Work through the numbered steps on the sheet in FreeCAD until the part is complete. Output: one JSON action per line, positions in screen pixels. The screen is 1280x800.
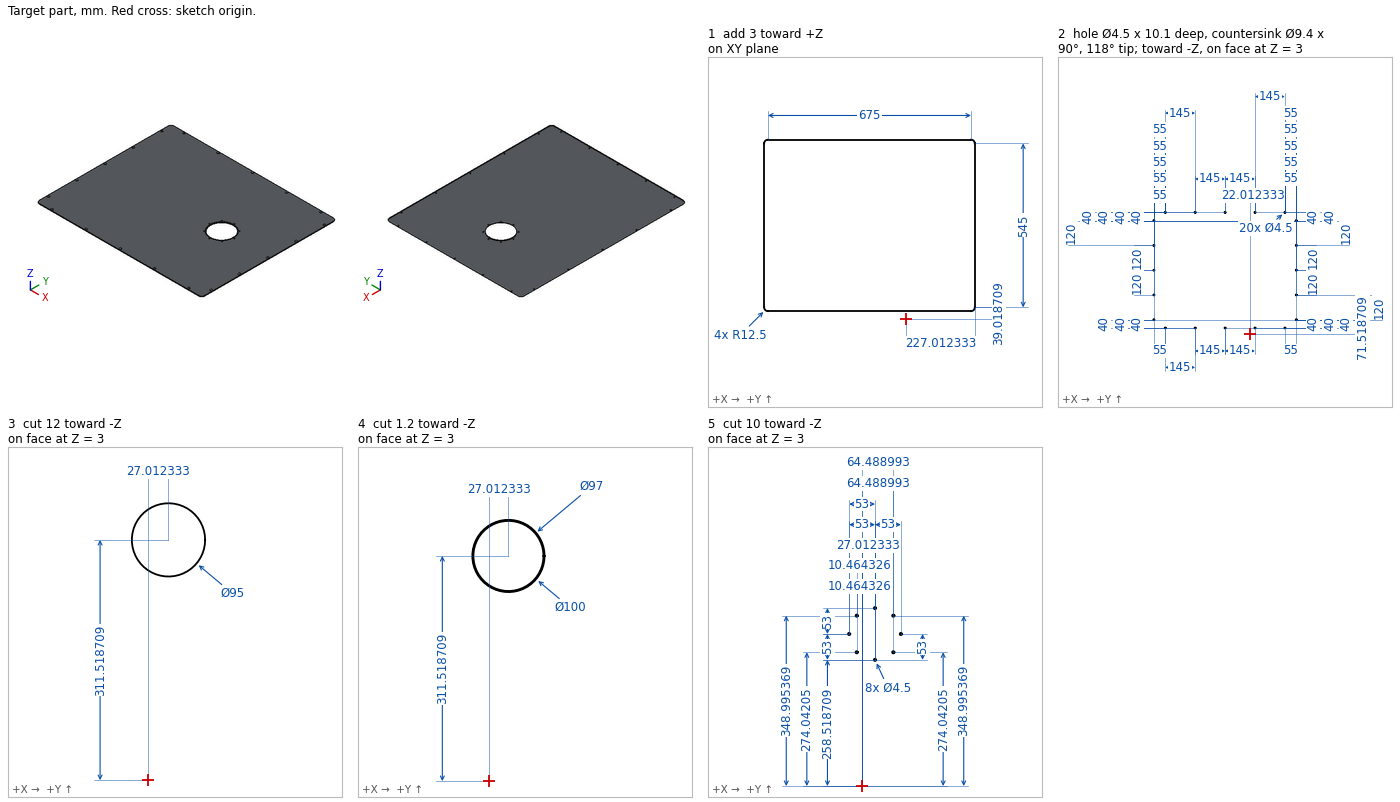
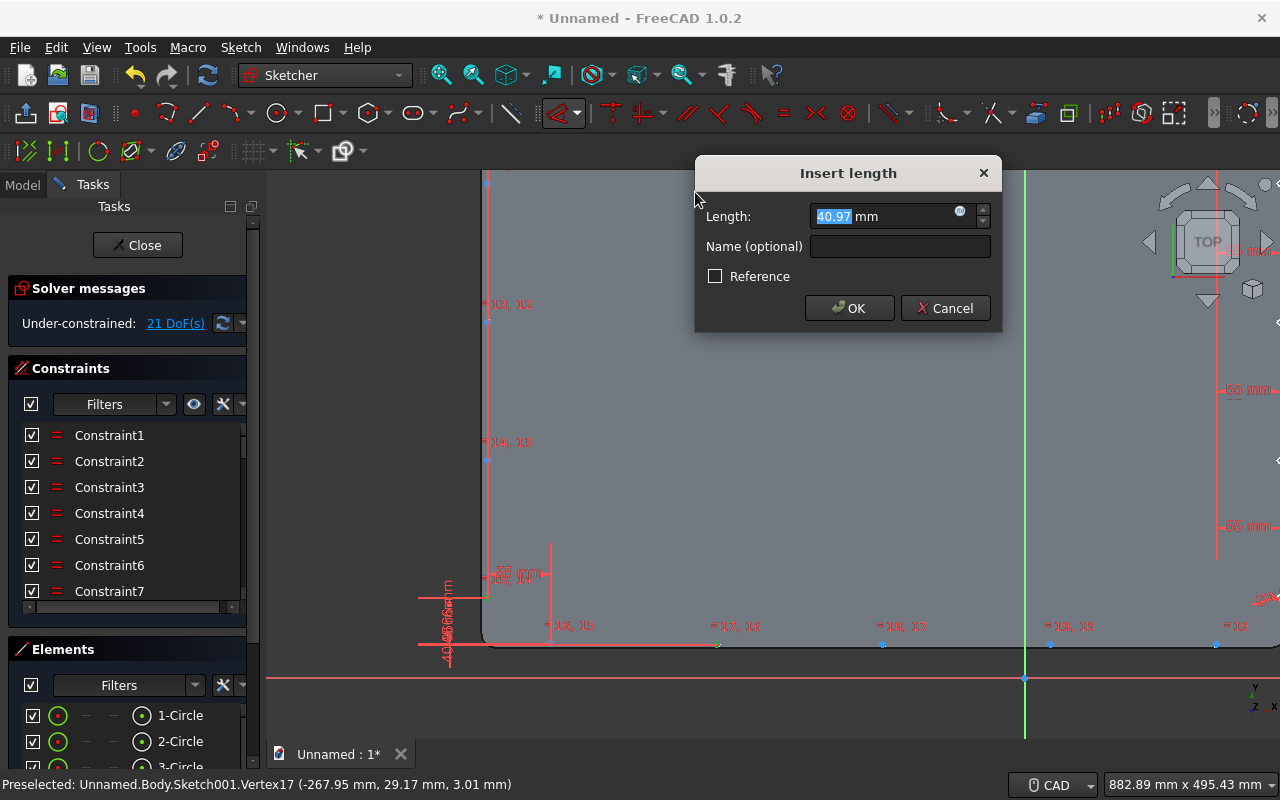
{"action": "type", "text": "40"}
{"action": "key", "text": "Return"}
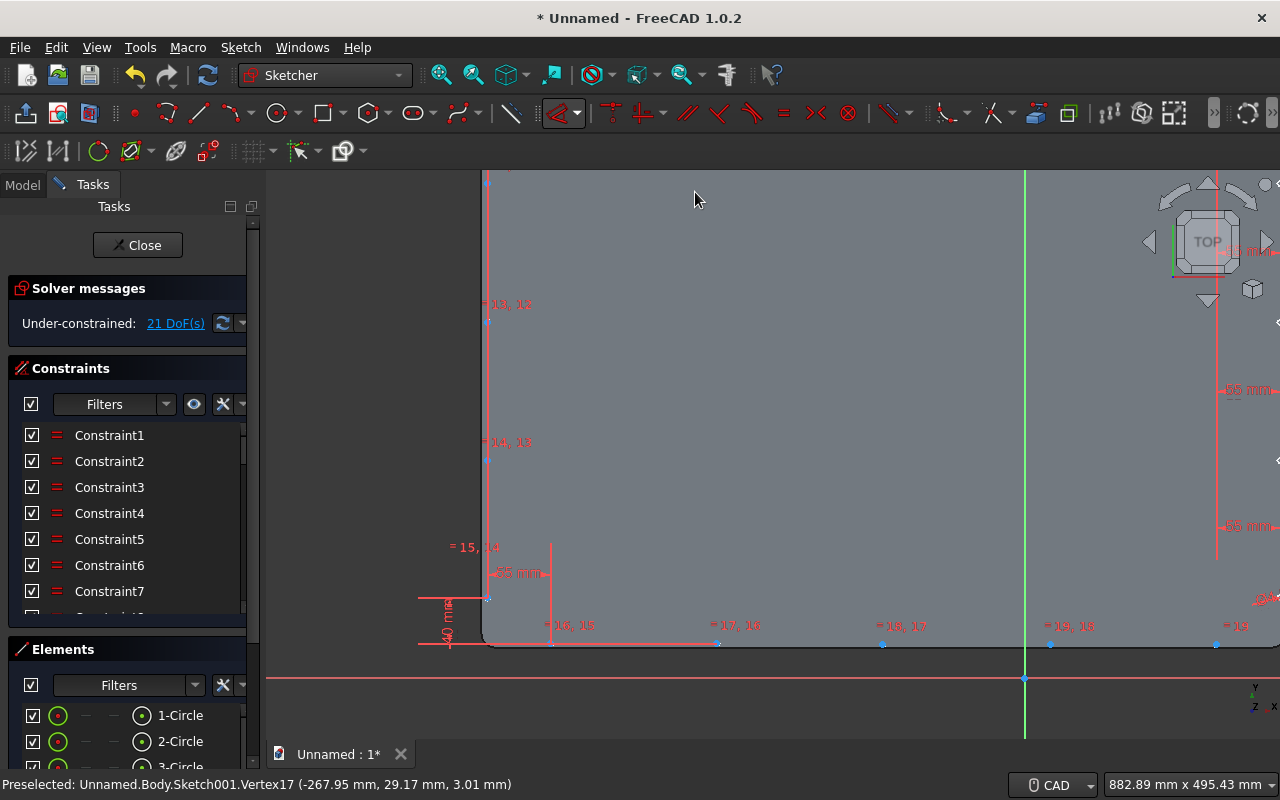
{"action": "scroll", "coordinate": [487, 597], "scroll_direction": "down", "scroll_amount": 3}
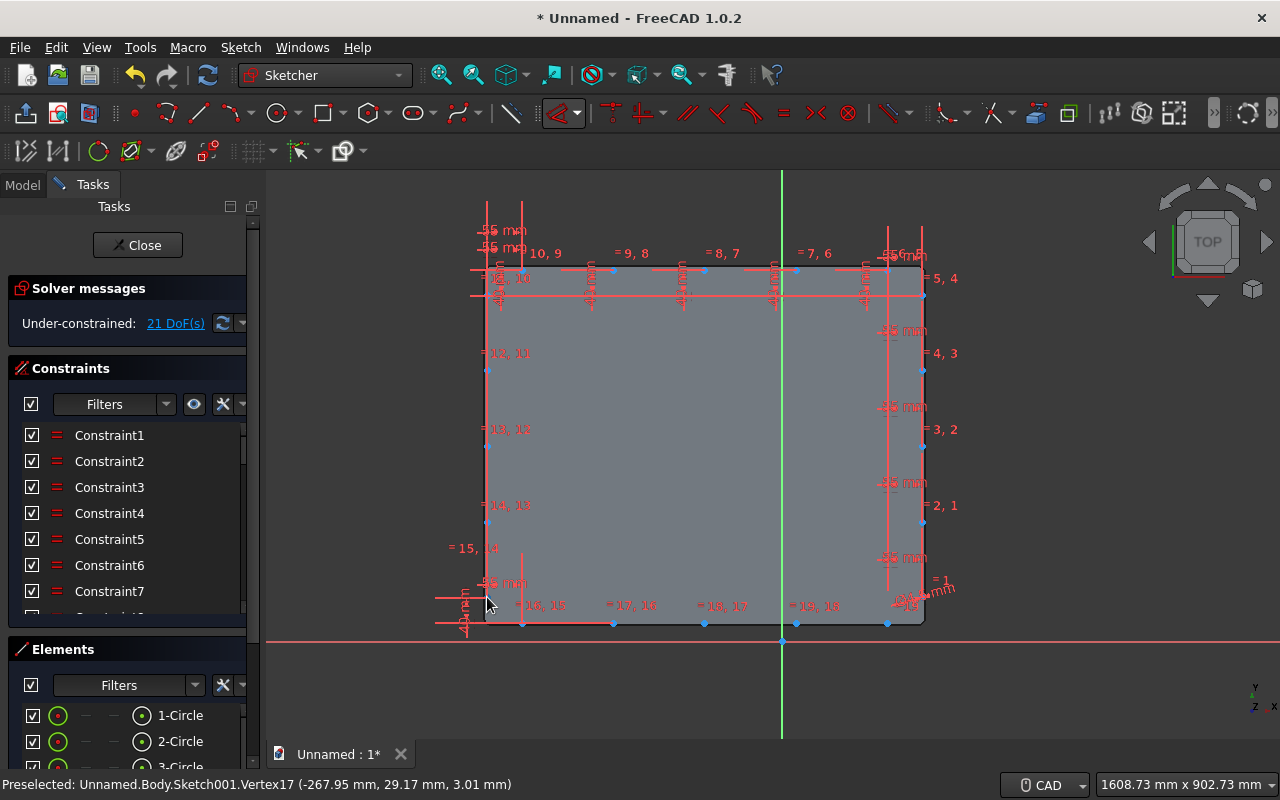
{"action": "scroll", "coordinate": [922, 597], "scroll_direction": "up", "scroll_amount": 3}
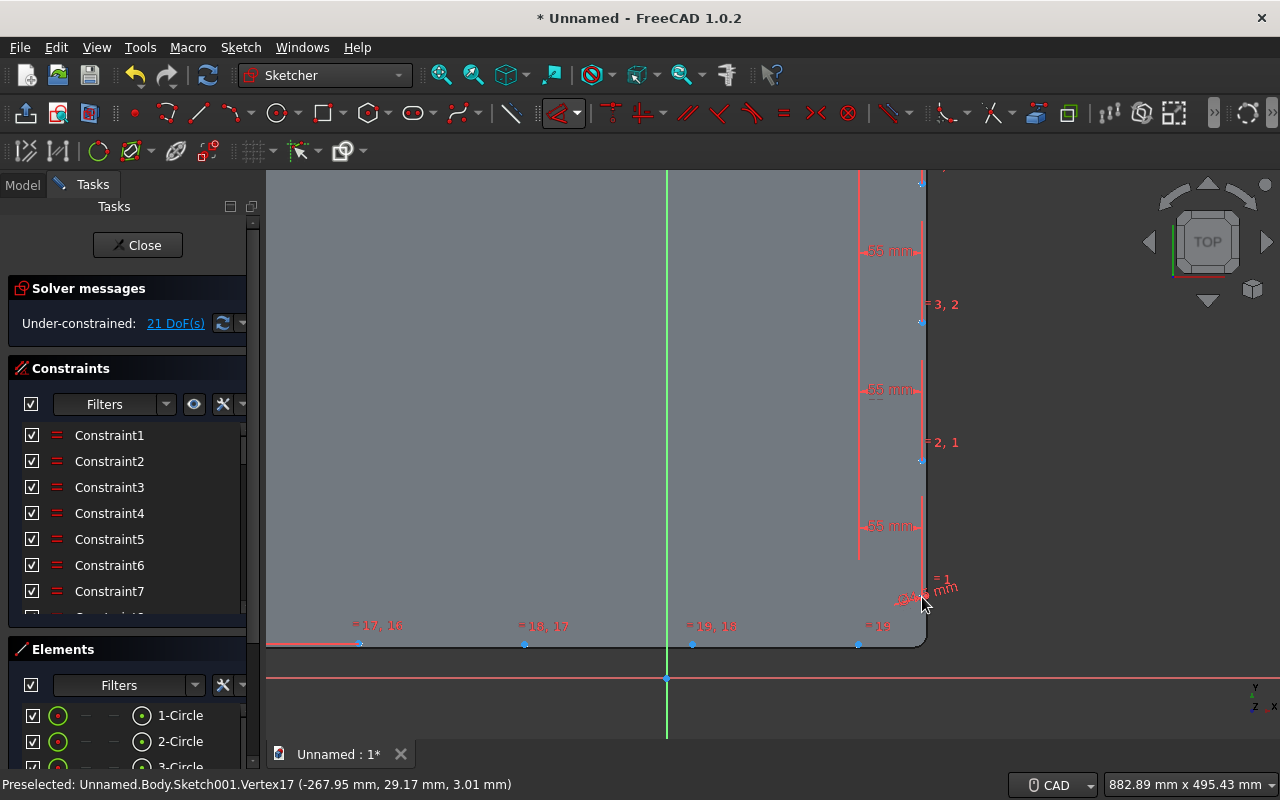
{"action": "left_click", "coordinate": [922, 597]}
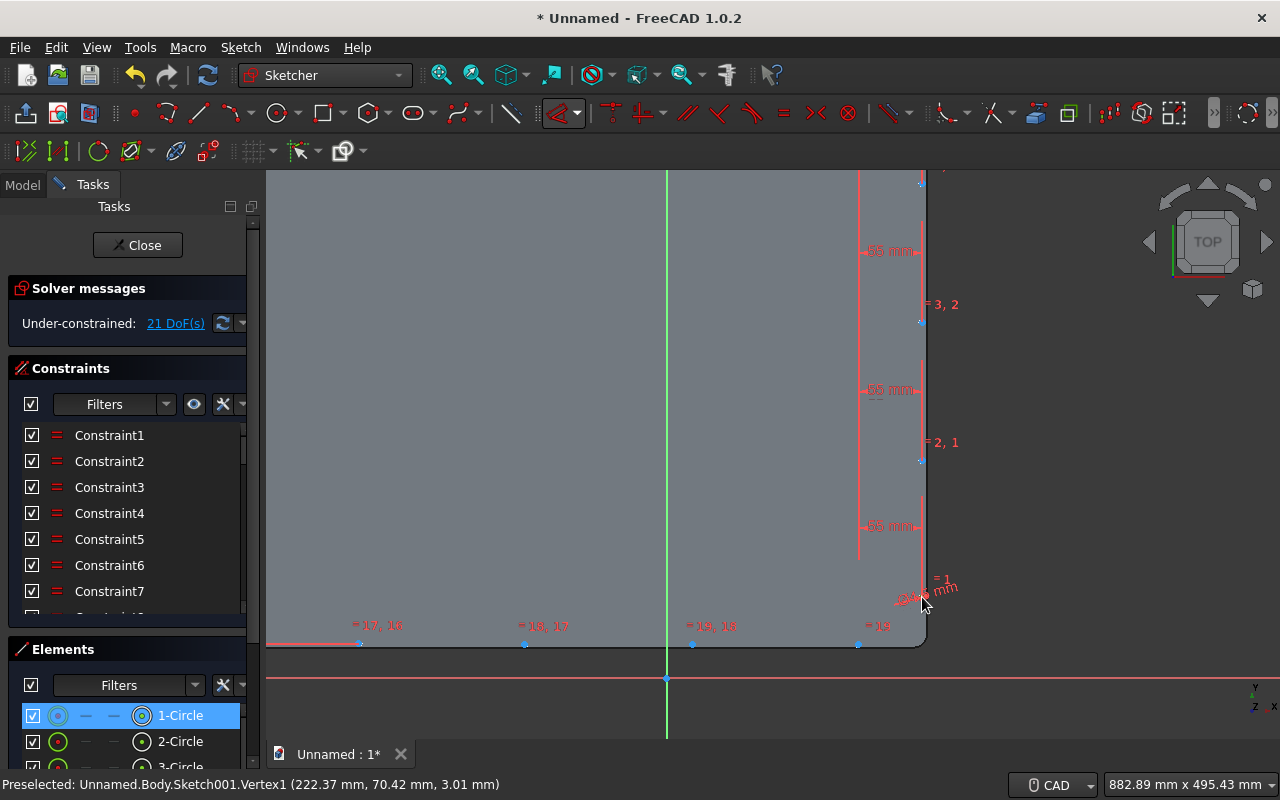
{"action": "left_click", "coordinate": [359, 644]}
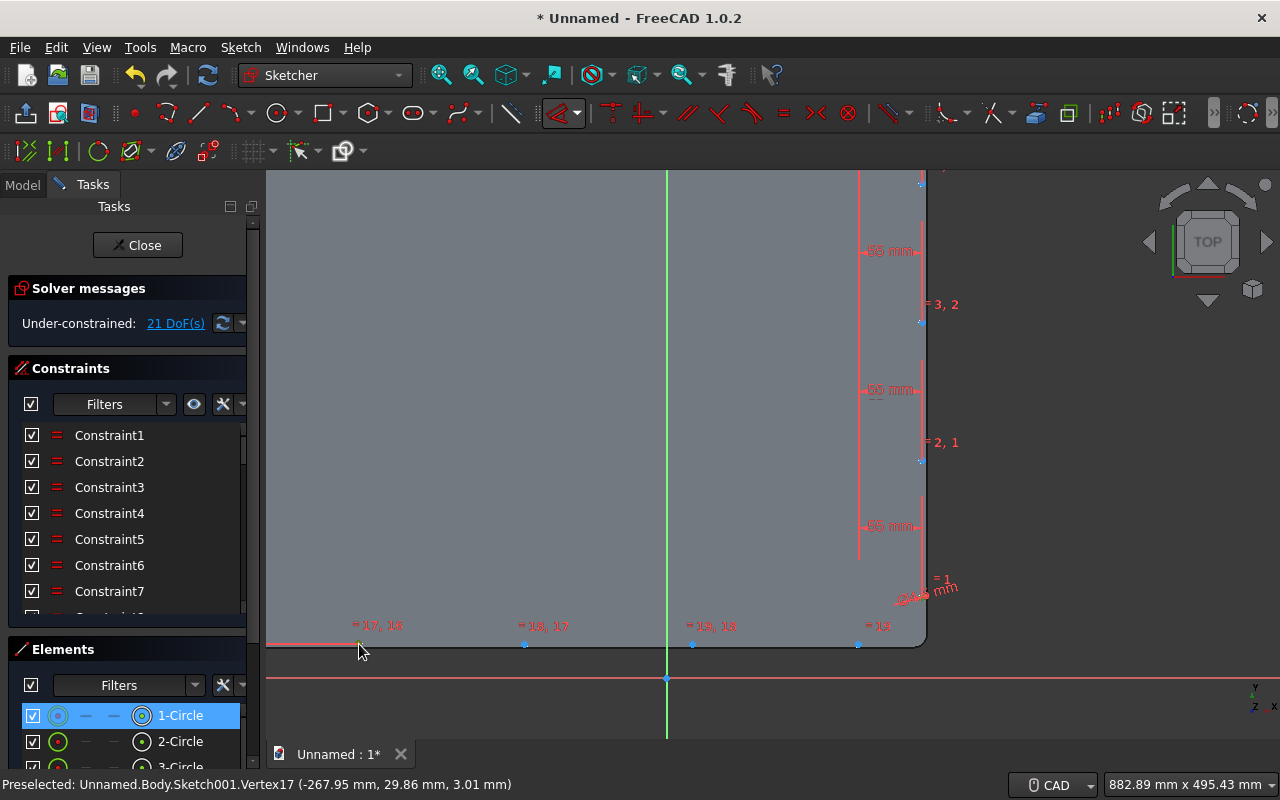
{"action": "key", "text": "i"}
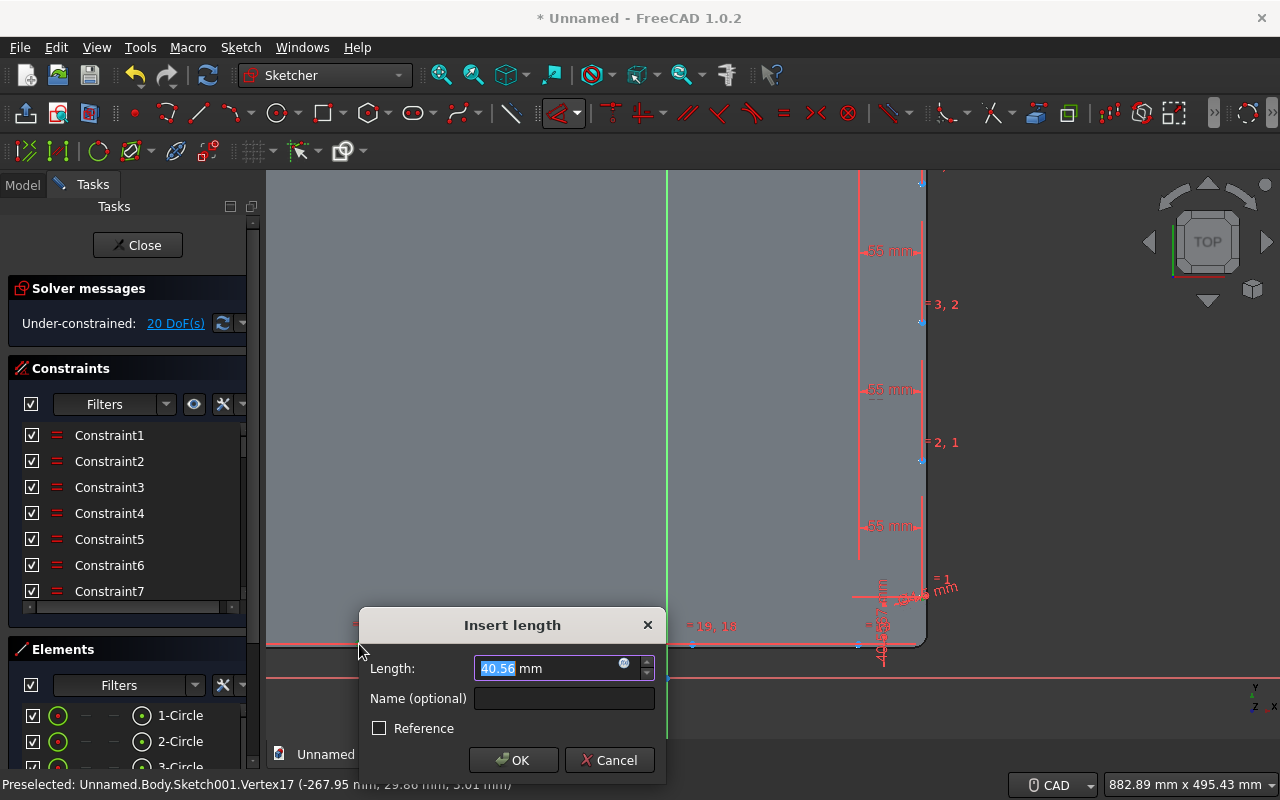
{"action": "type", "text": "40"}
{"action": "key", "text": "Return"}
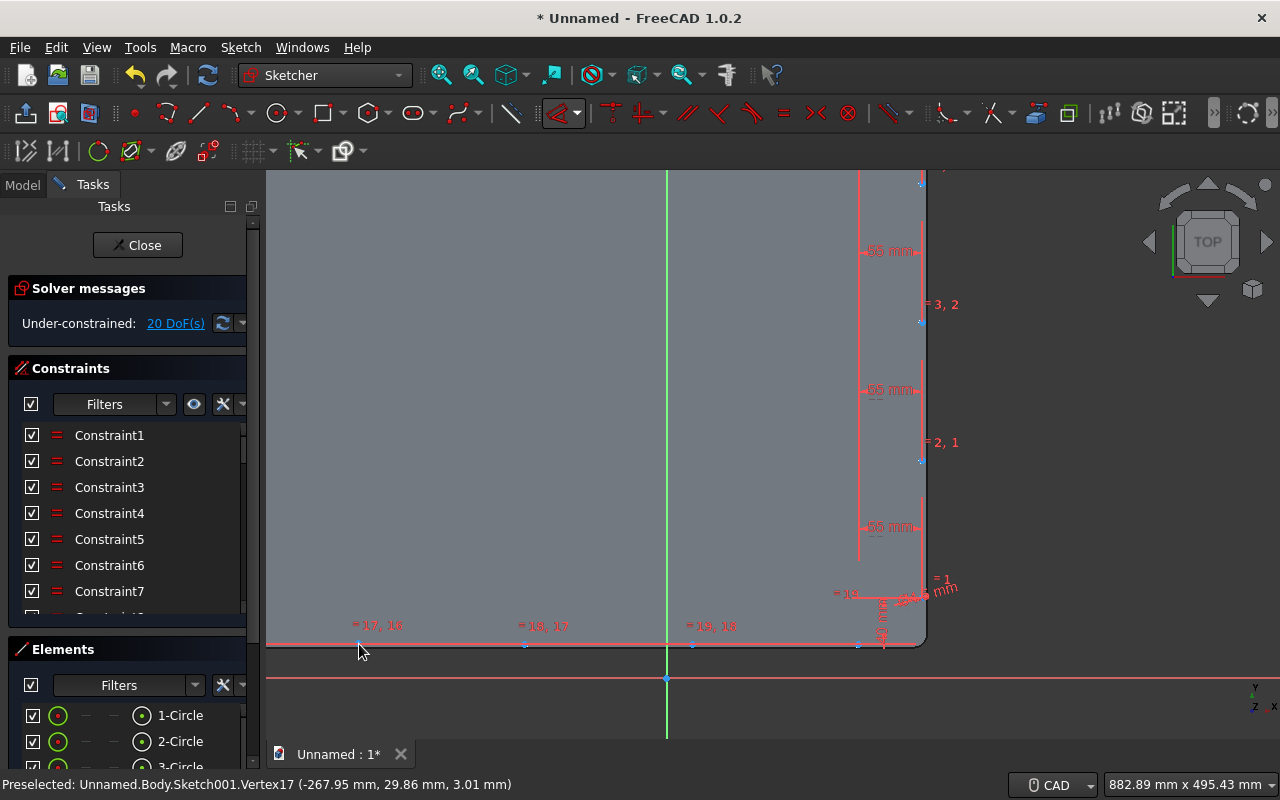
{"action": "left_click", "coordinate": [922, 598]}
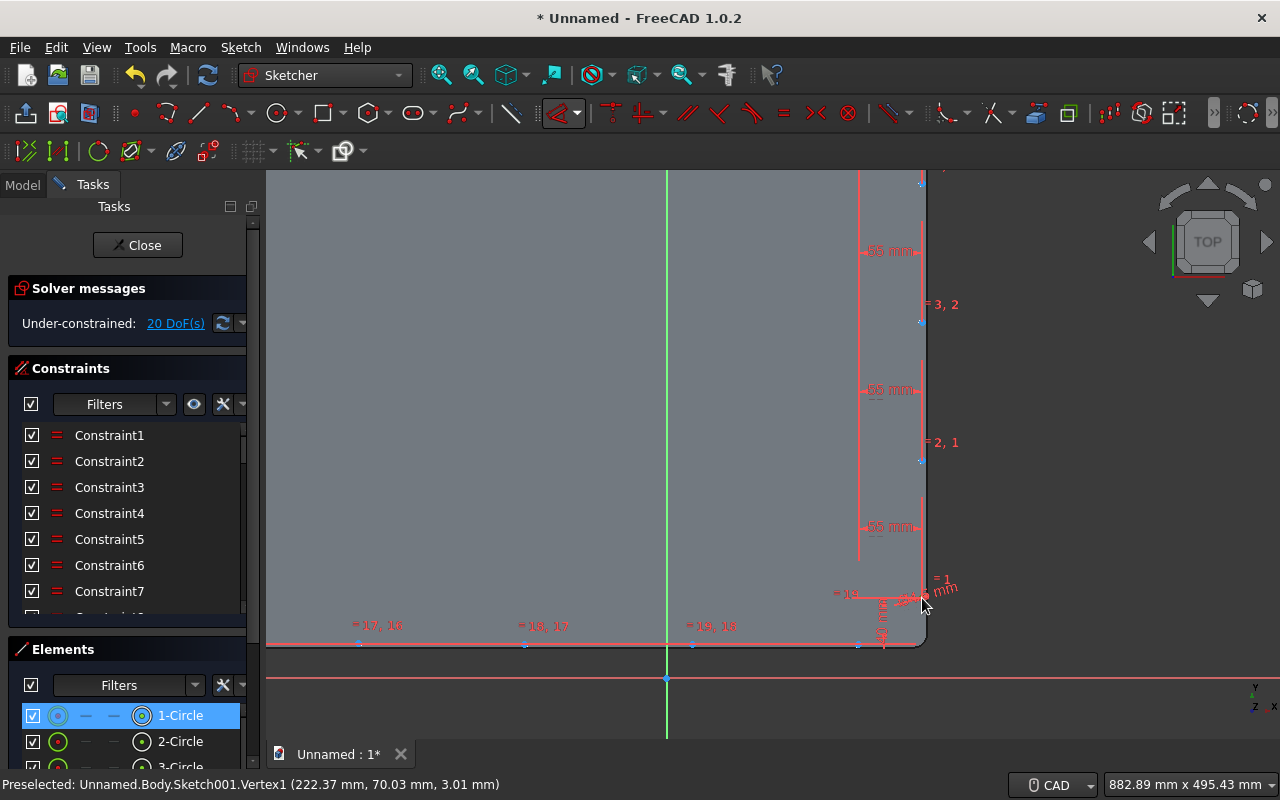
{"action": "left_click", "coordinate": [525, 645]}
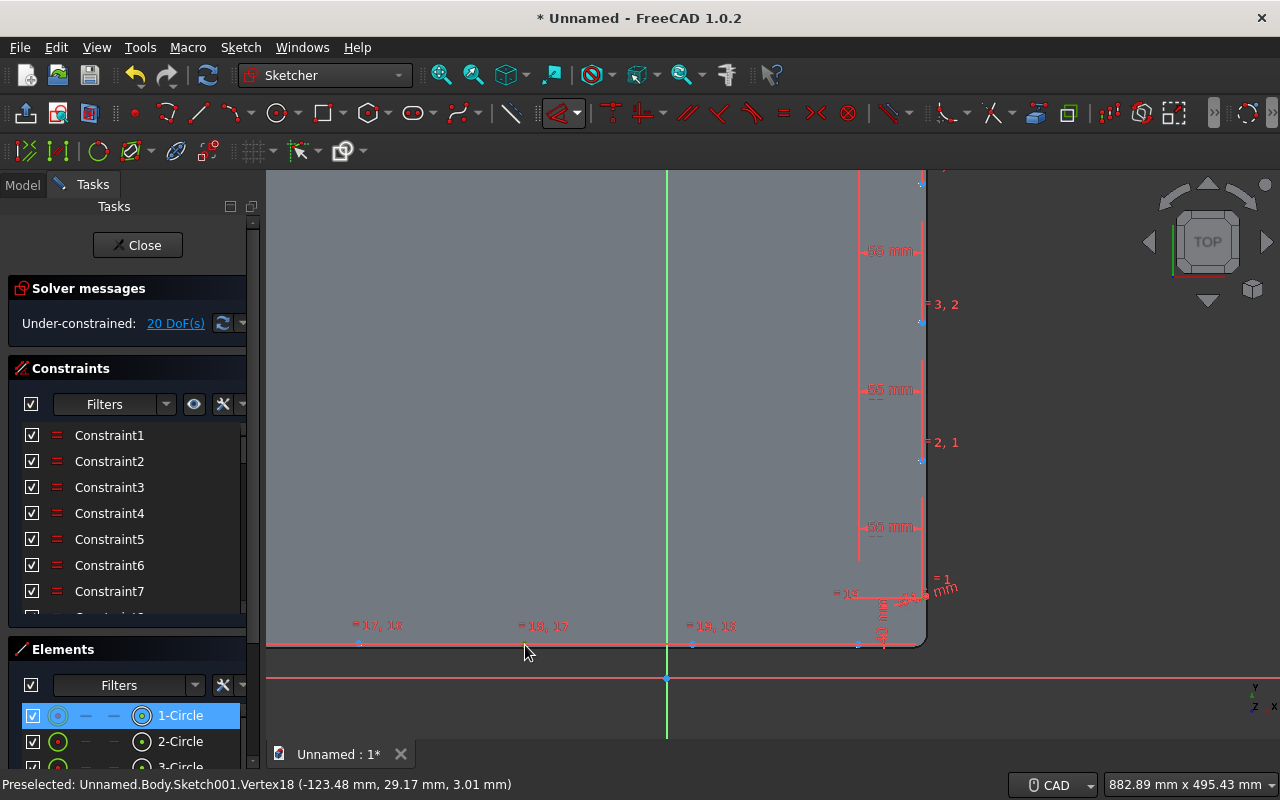
{"action": "key", "text": "i"}